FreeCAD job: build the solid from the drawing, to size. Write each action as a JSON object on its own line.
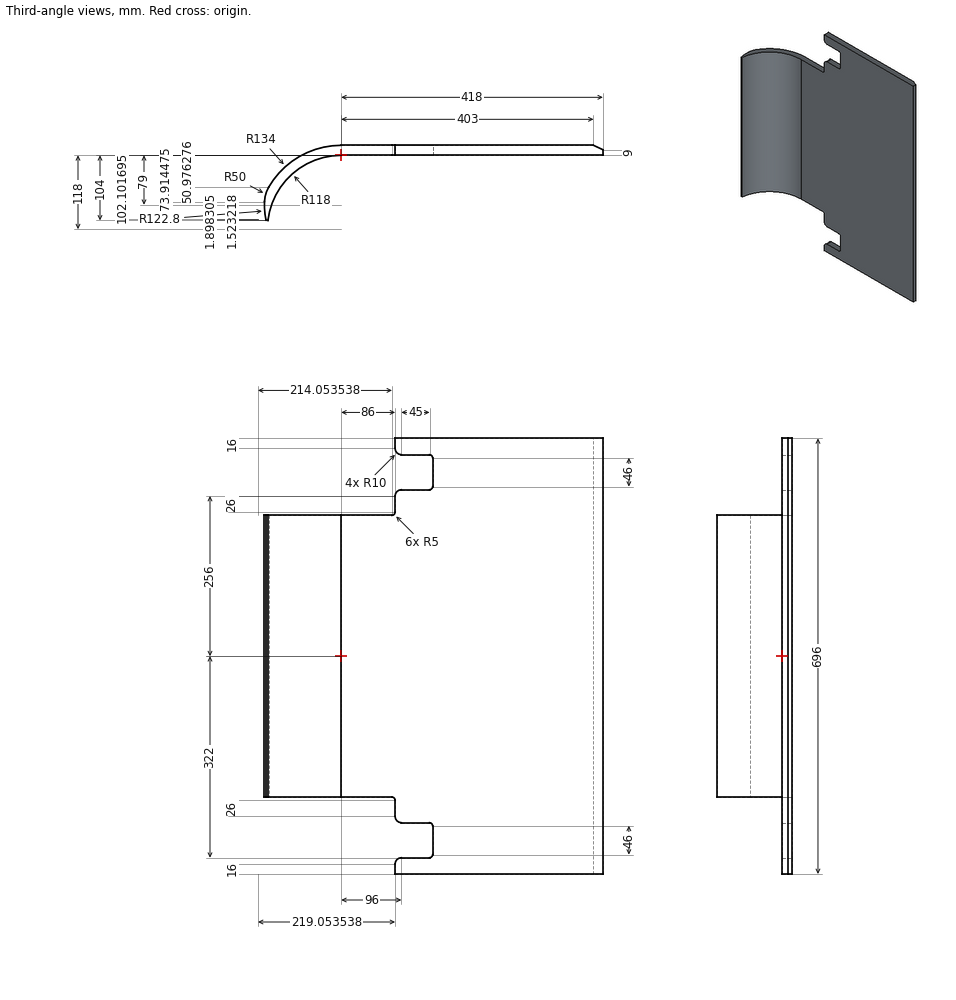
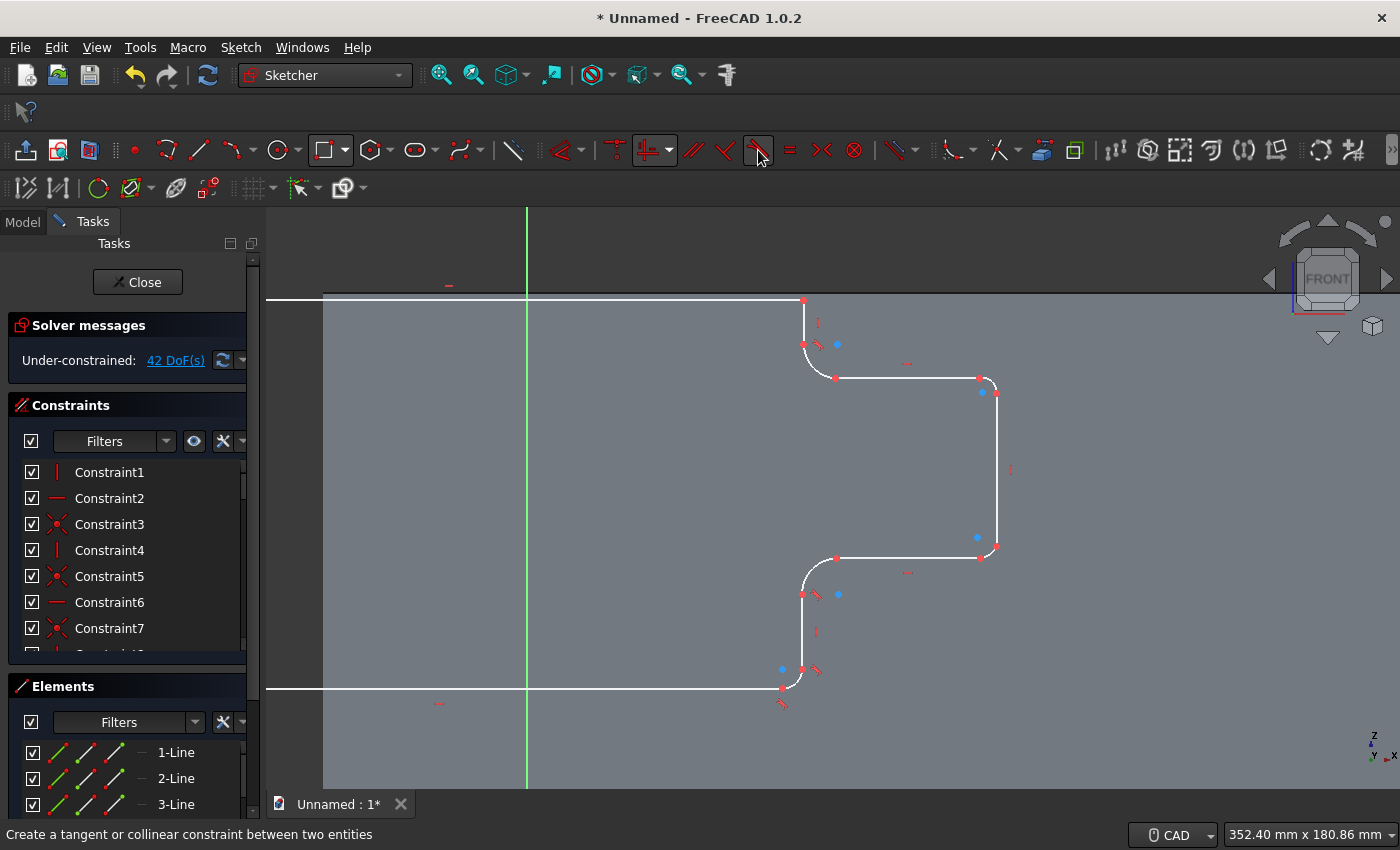
{"action": "scroll", "coordinate": [807, 317], "scroll_direction": "down", "scroll_amount": 9}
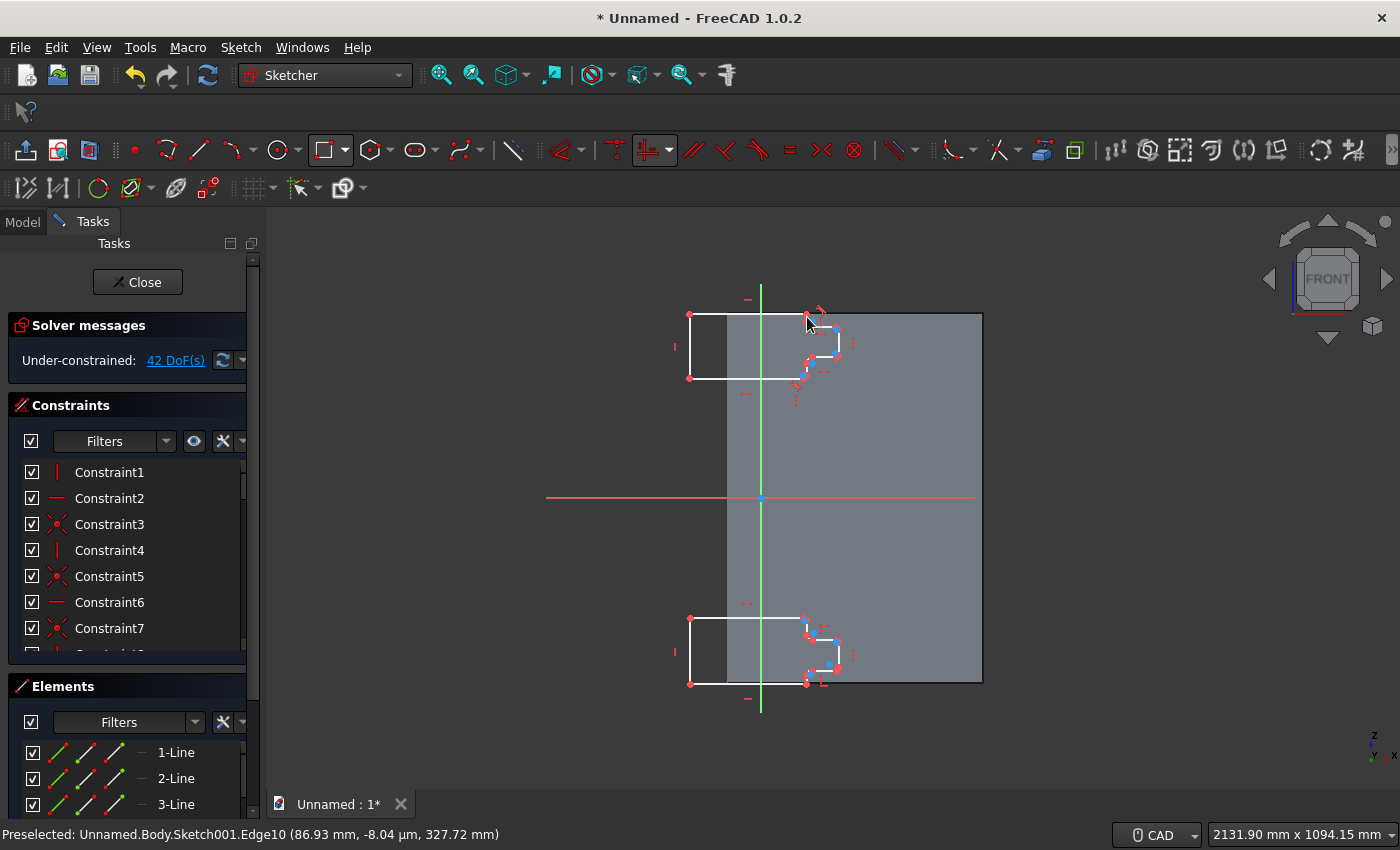
{"action": "scroll", "coordinate": [819, 327], "scroll_direction": "up", "scroll_amount": 4}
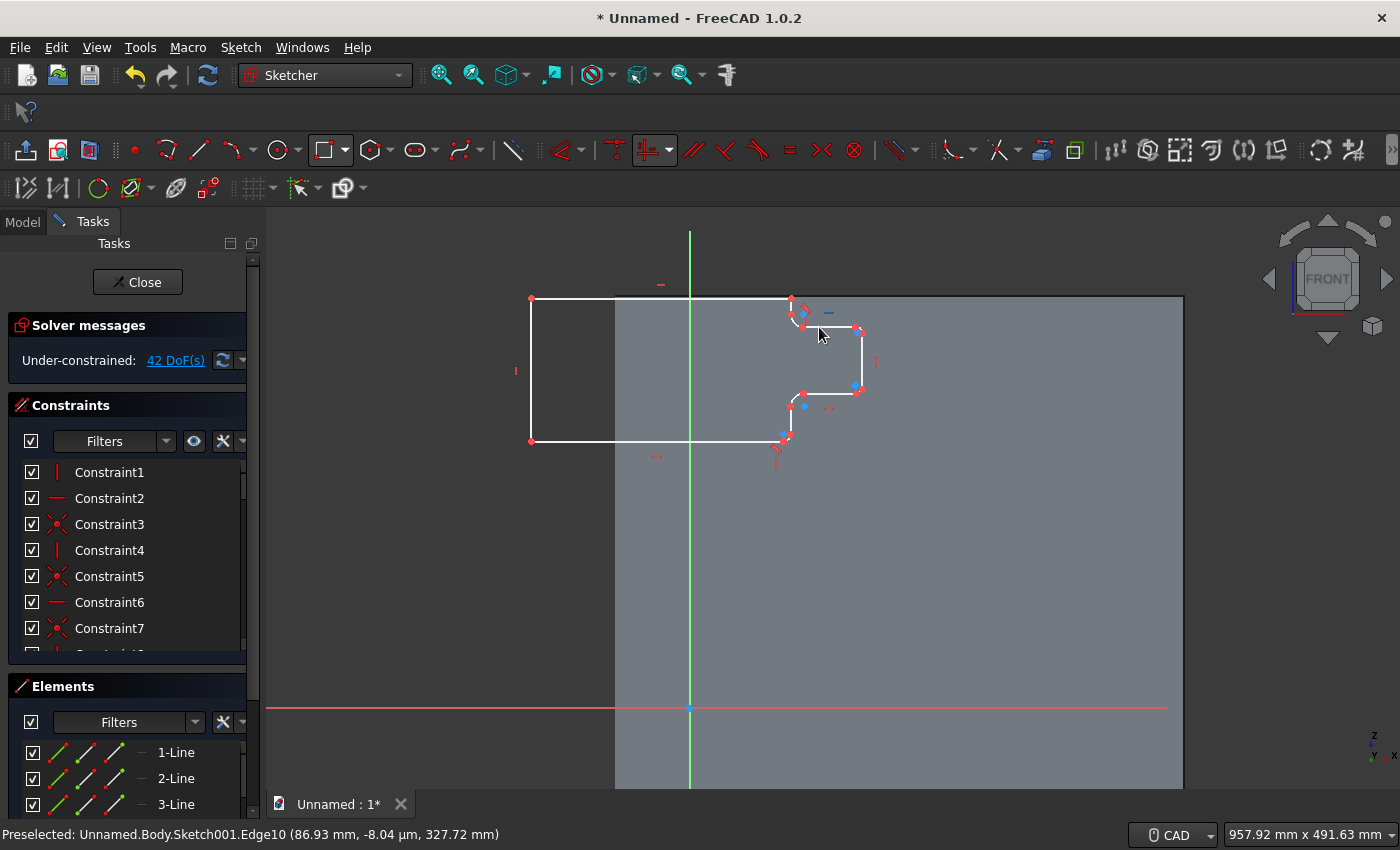
{"action": "left_click", "coordinate": [819, 327]}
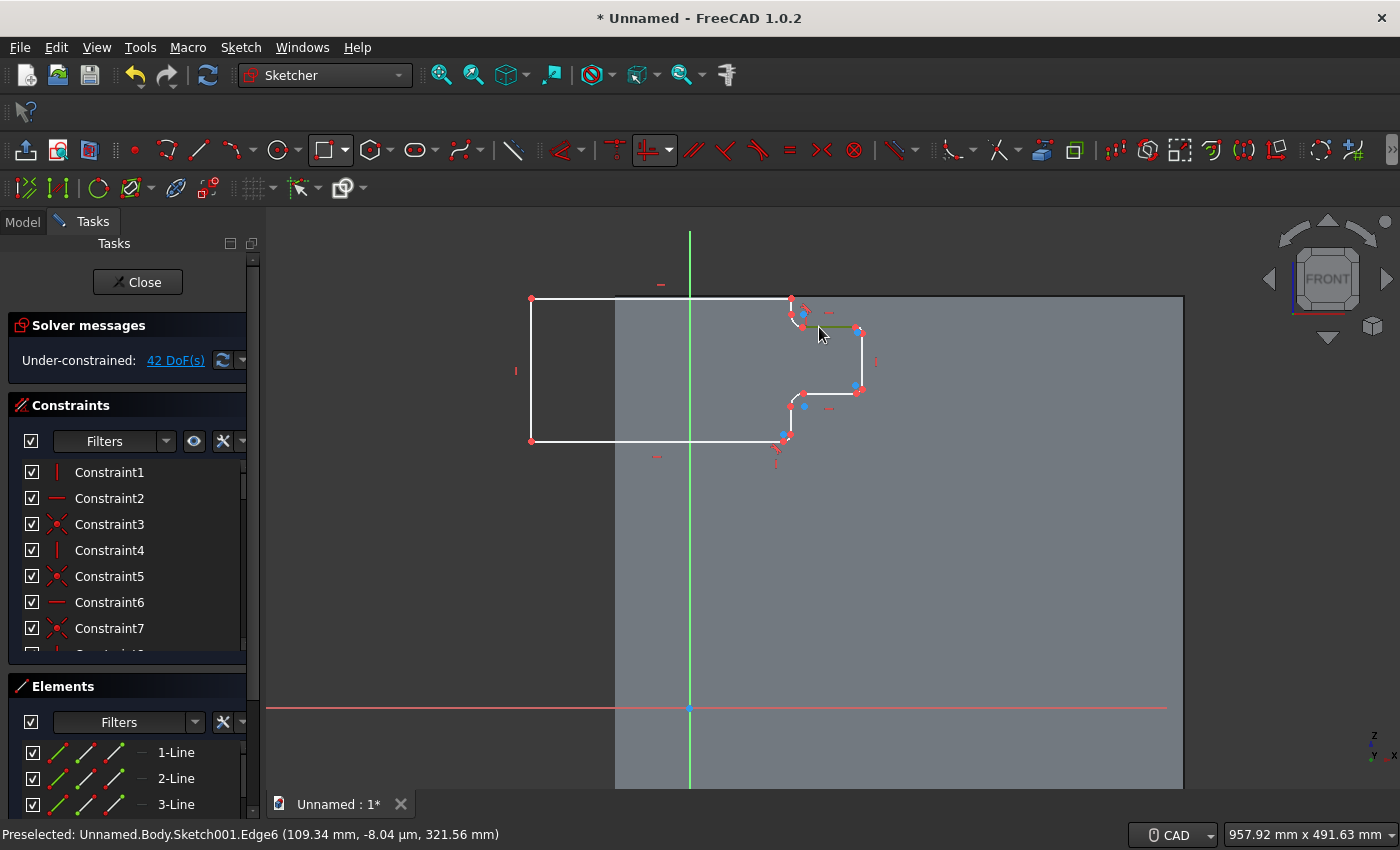
{"action": "scroll", "coordinate": [795, 323], "scroll_direction": "up", "scroll_amount": 3}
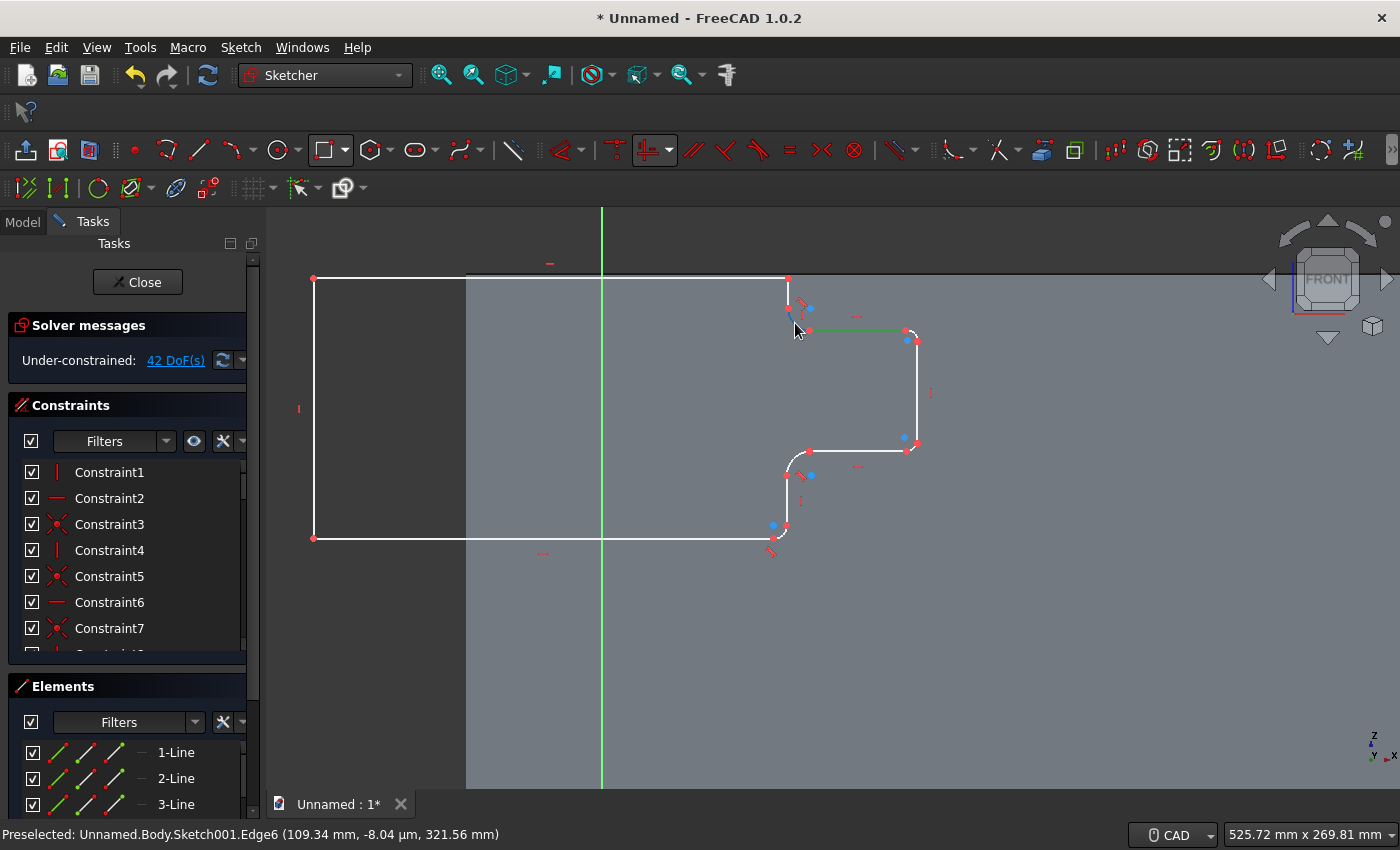
{"action": "left_click", "coordinate": [794, 324]}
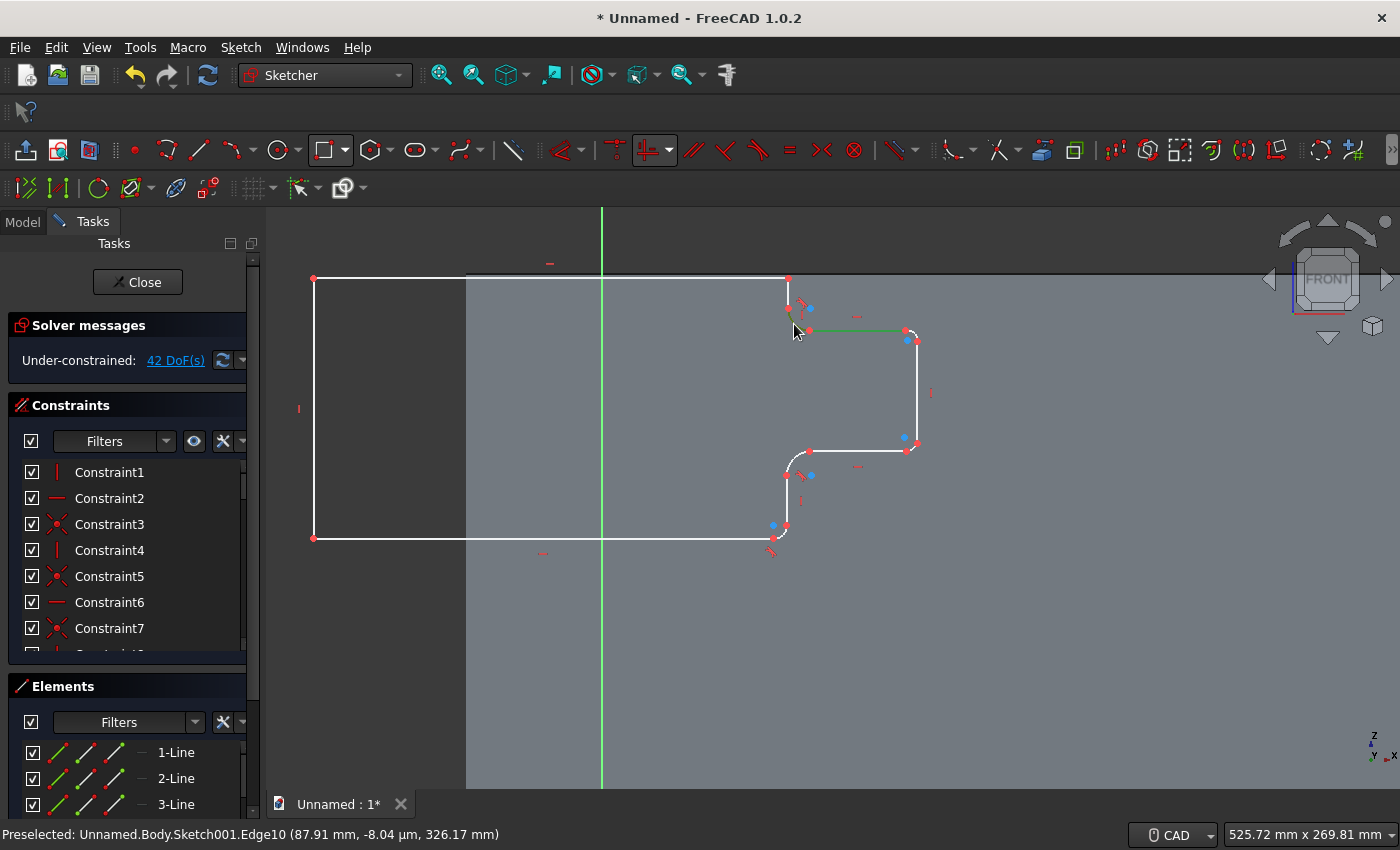
{"action": "left_click", "coordinate": [758, 150]}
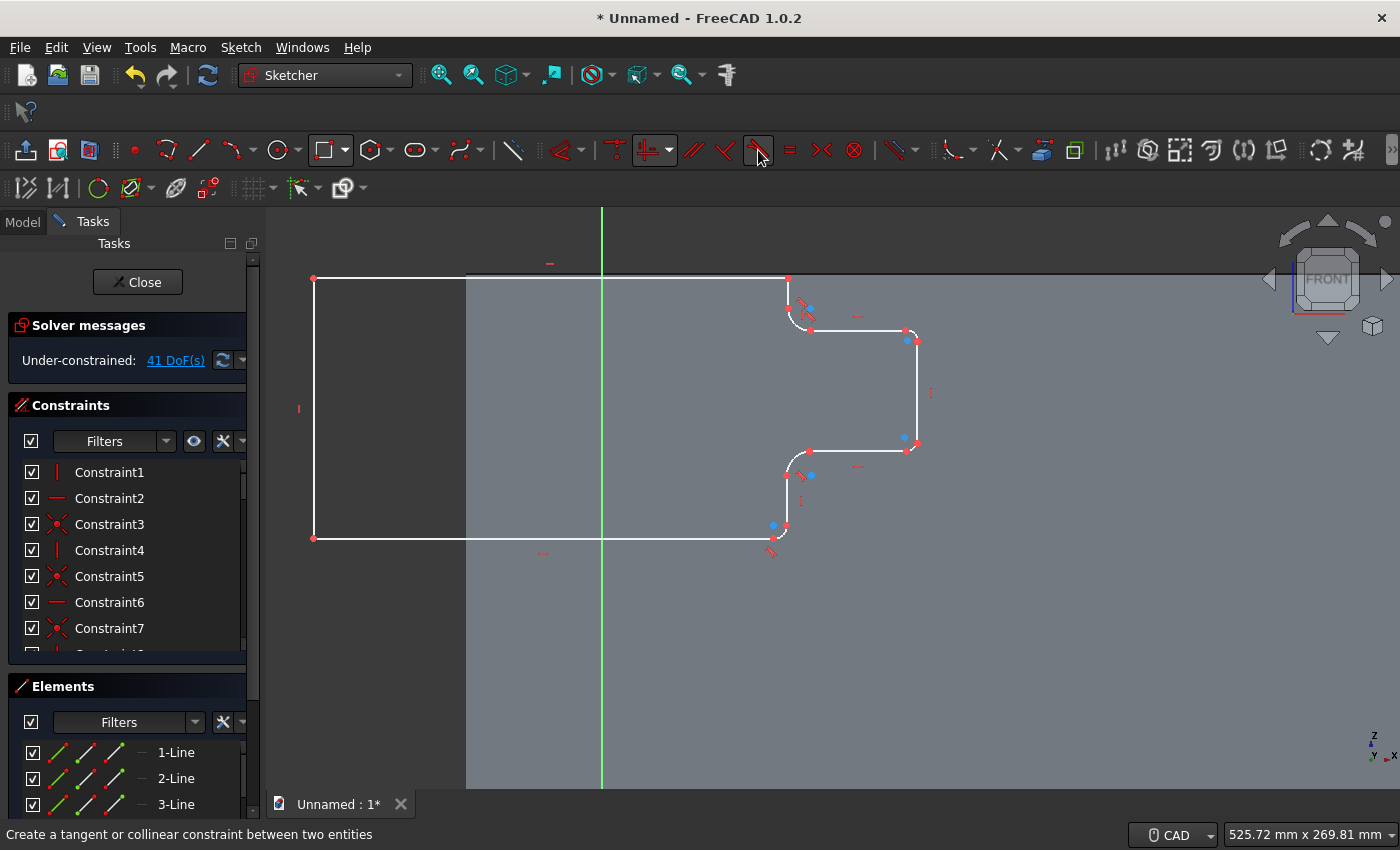
{"action": "left_click", "coordinate": [839, 331]}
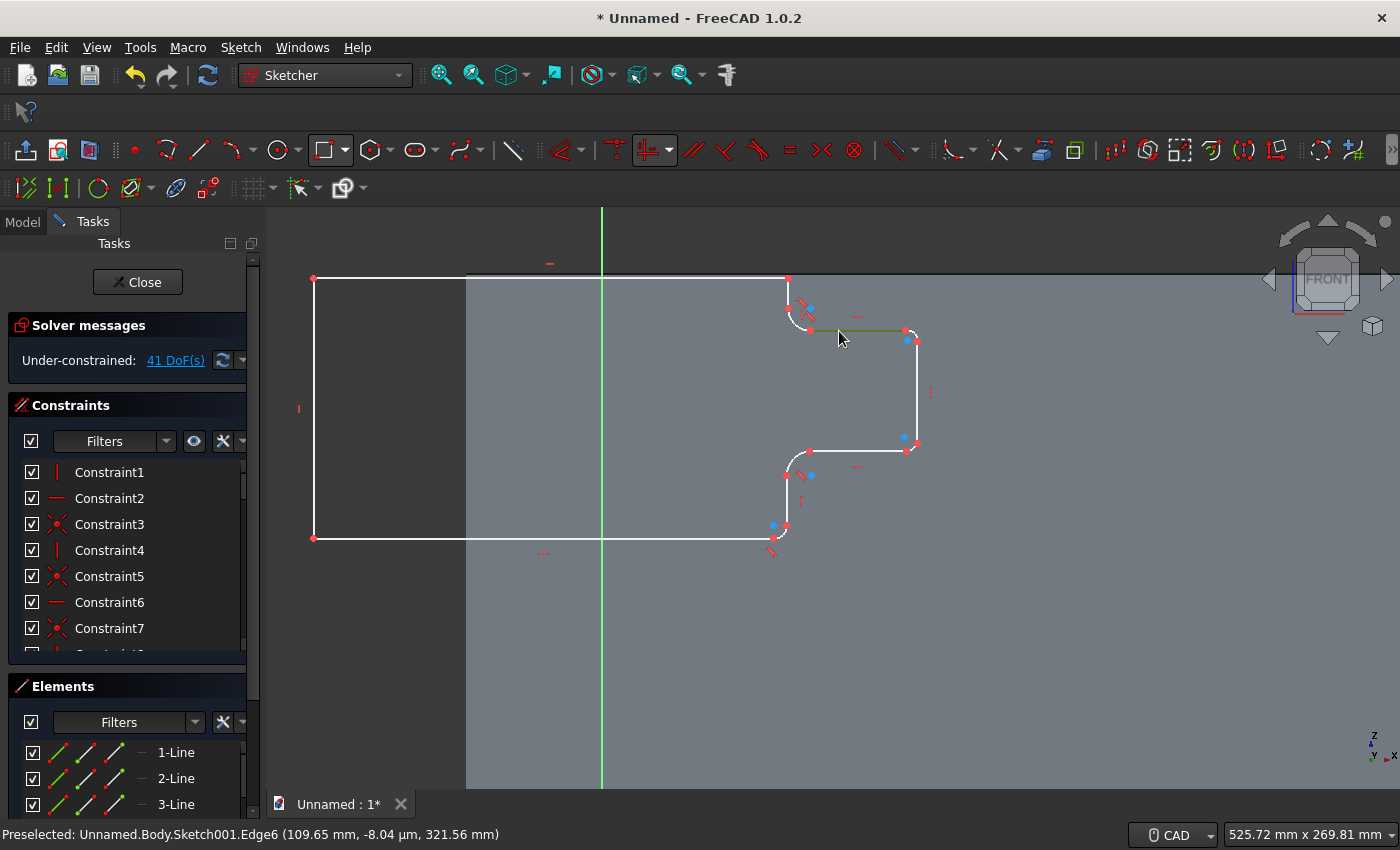
{"action": "scroll", "coordinate": [914, 333], "scroll_direction": "up", "scroll_amount": 3}